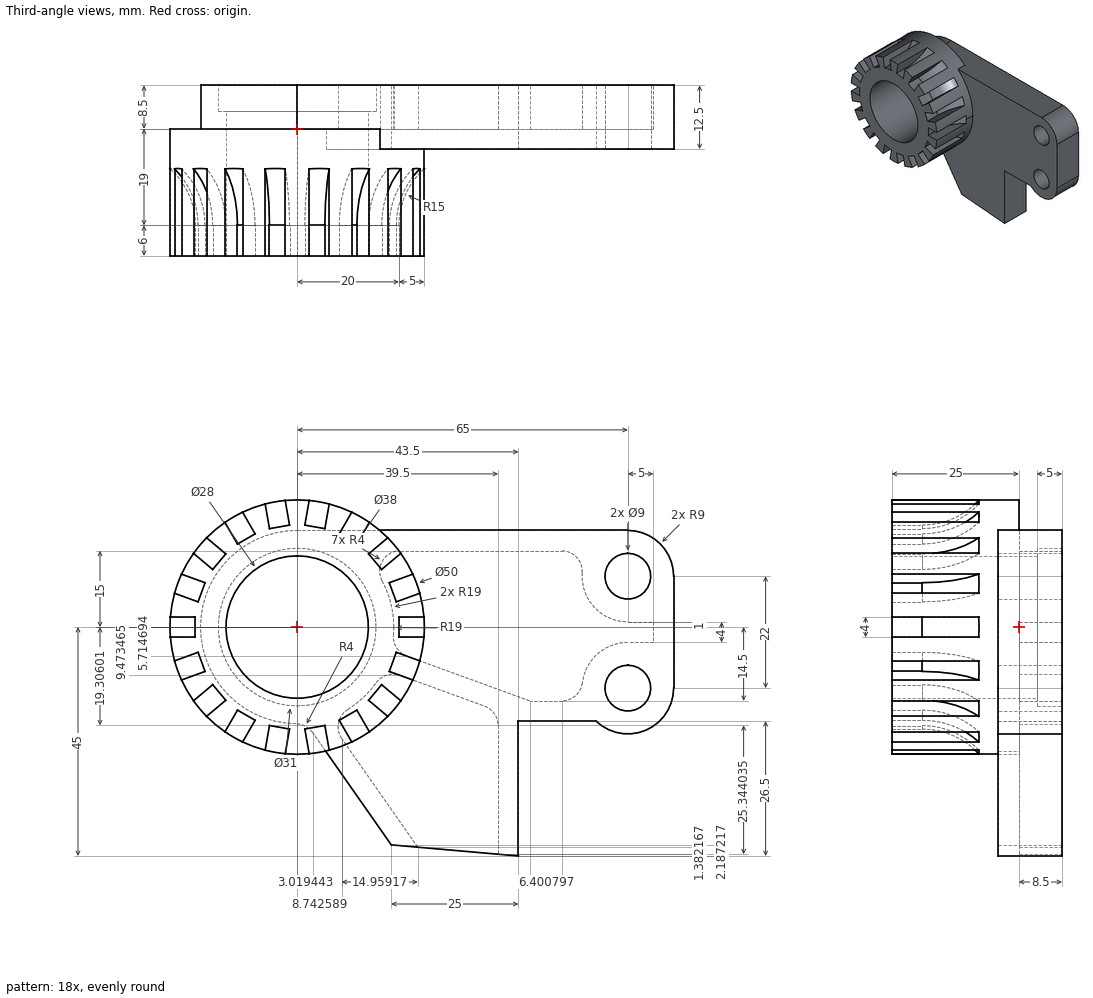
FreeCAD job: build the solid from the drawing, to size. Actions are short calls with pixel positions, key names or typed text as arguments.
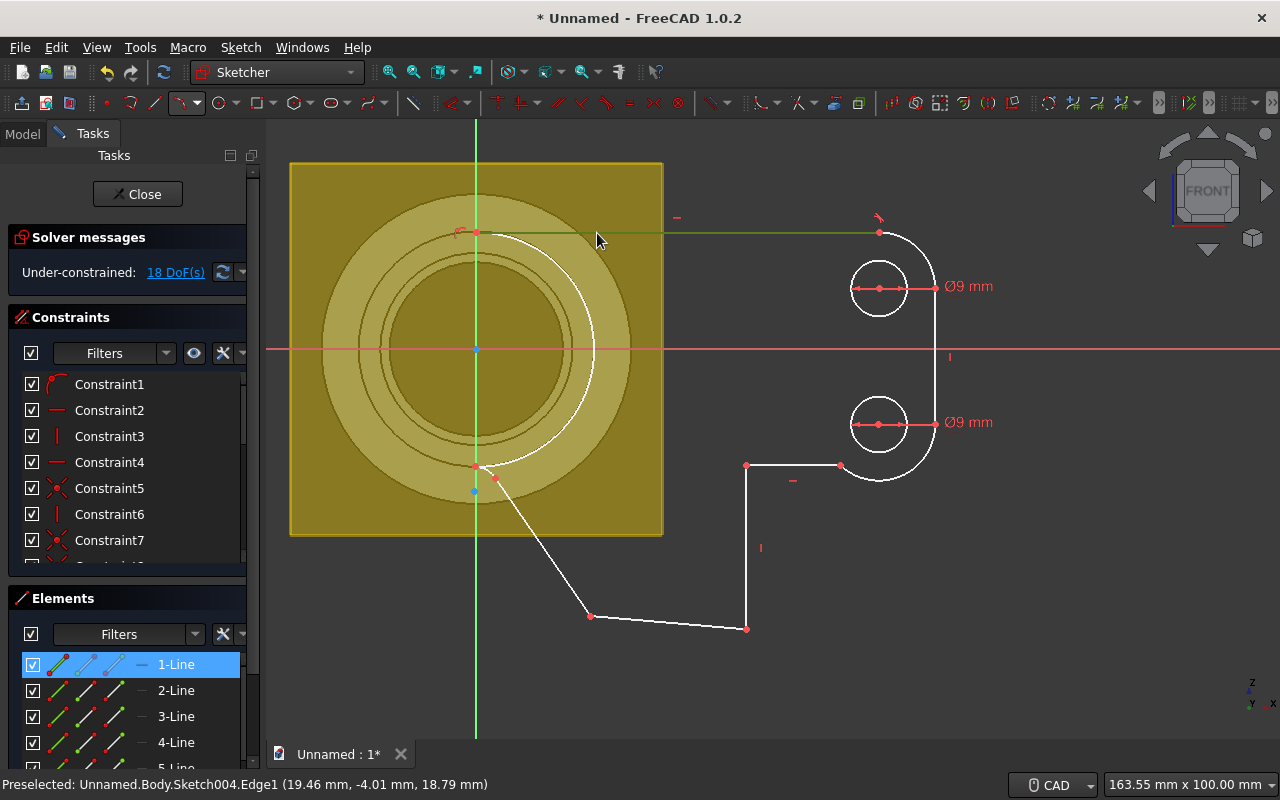
click(571, 420)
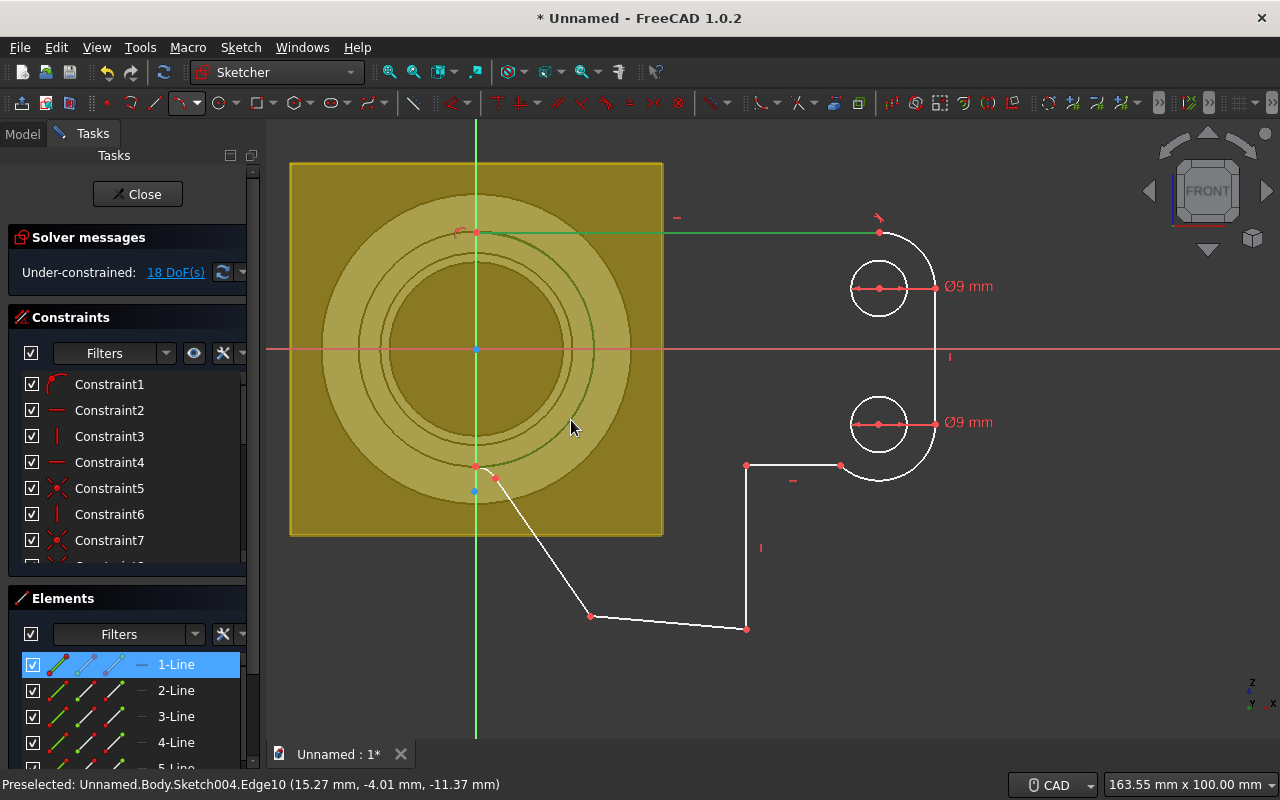
click(606, 104)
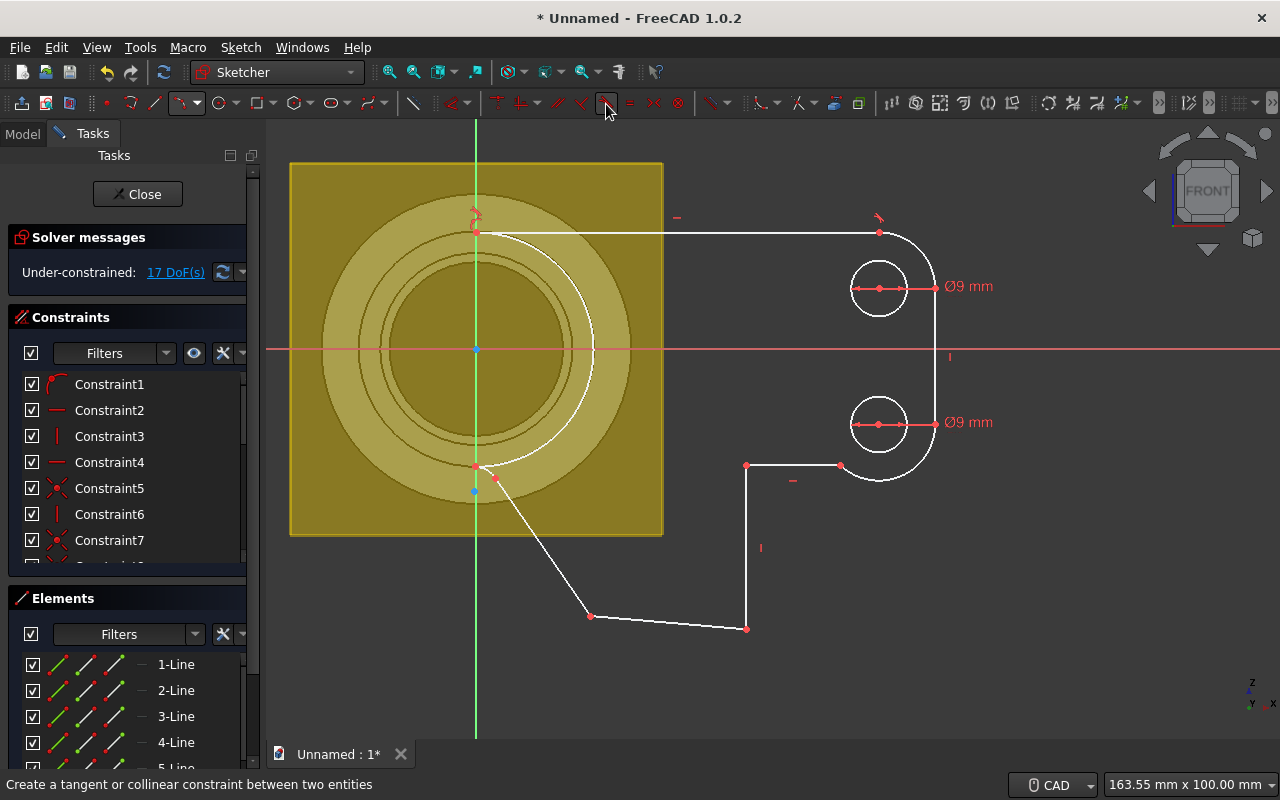
click(935, 329)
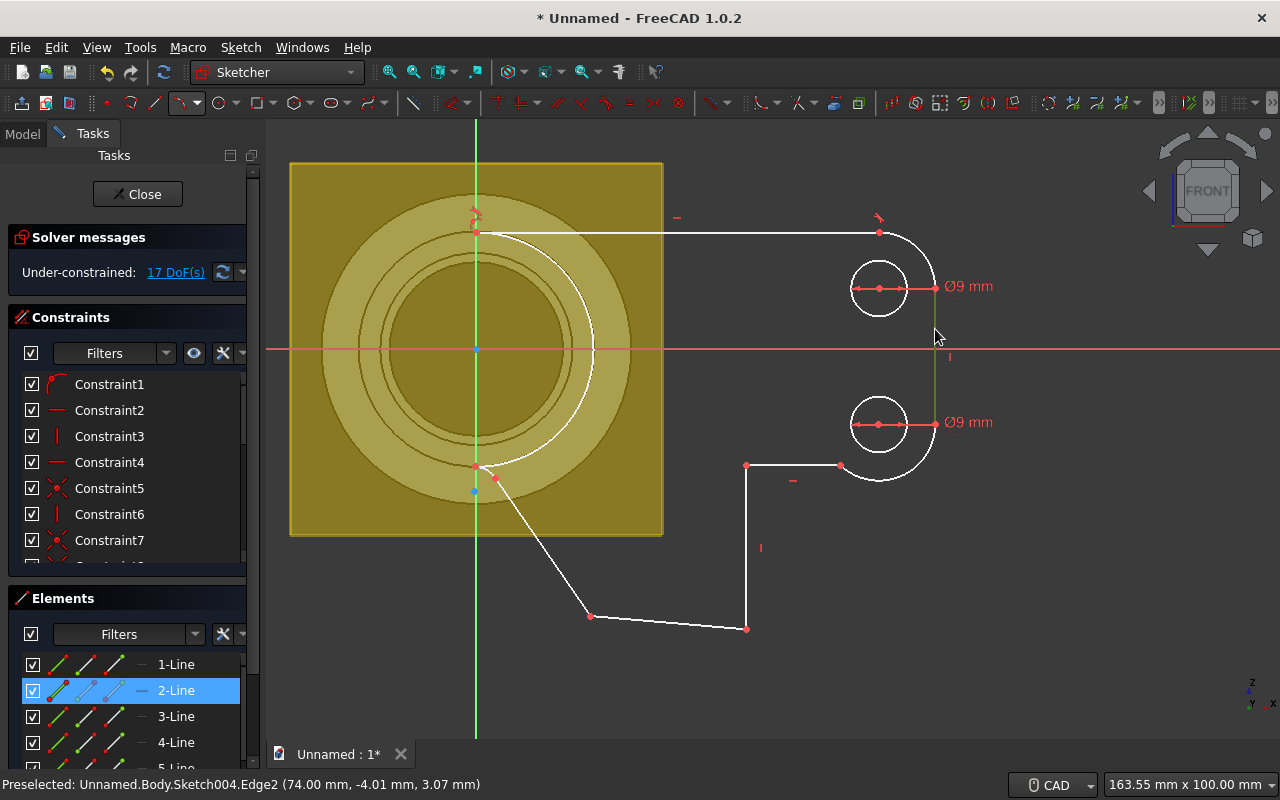
click(929, 263)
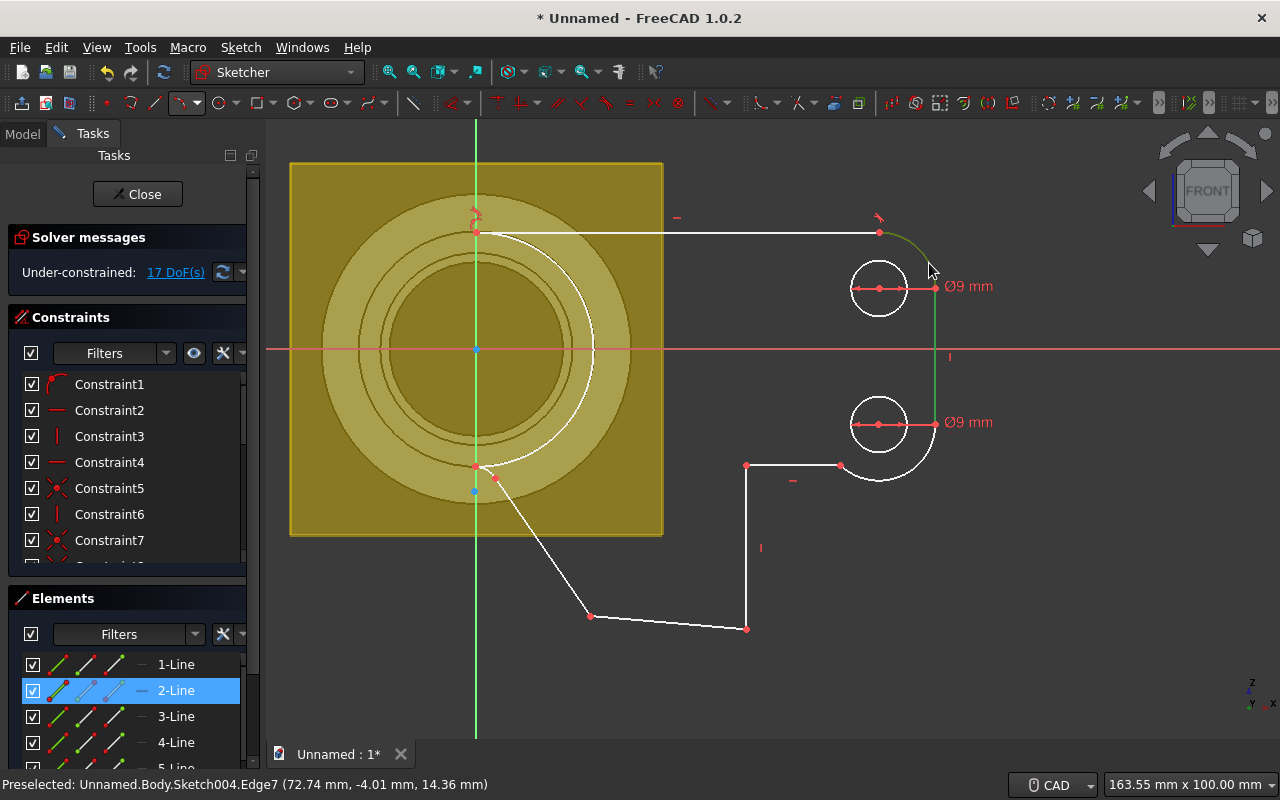
click(606, 104)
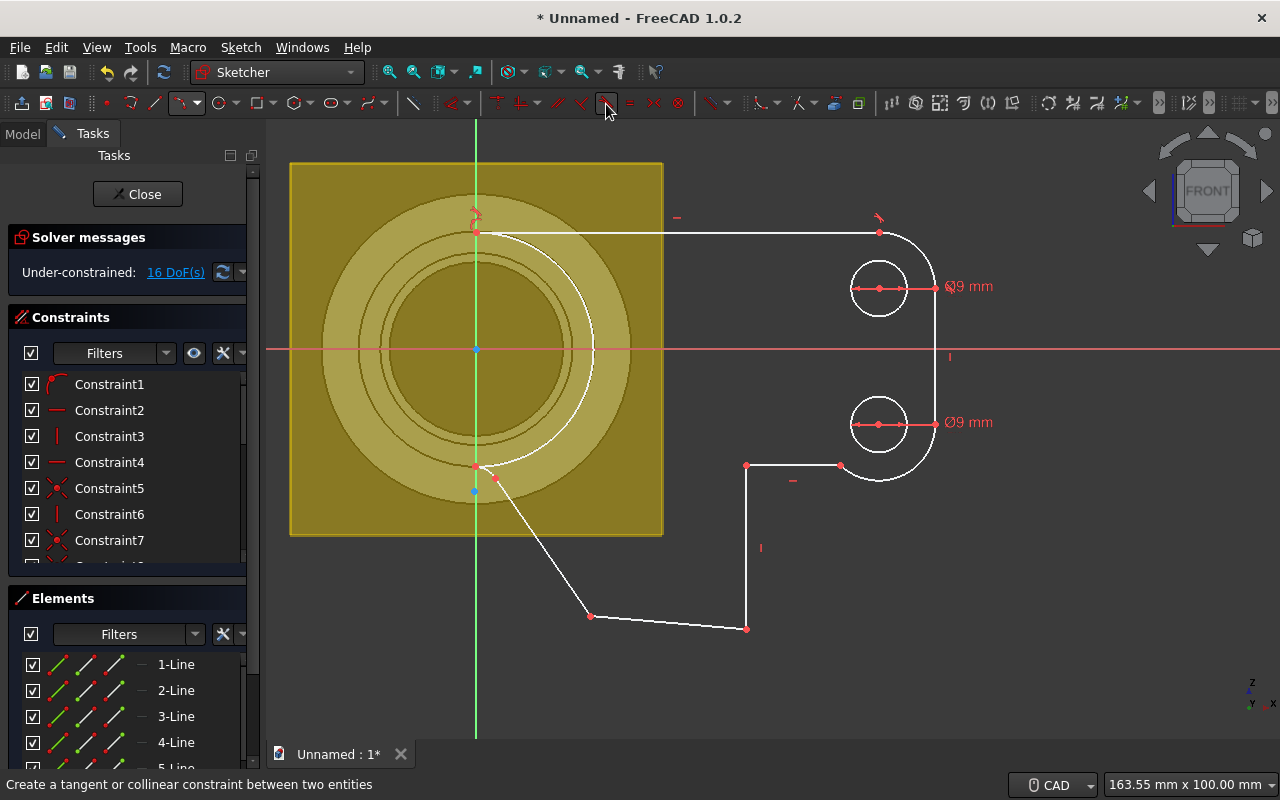
click(935, 329)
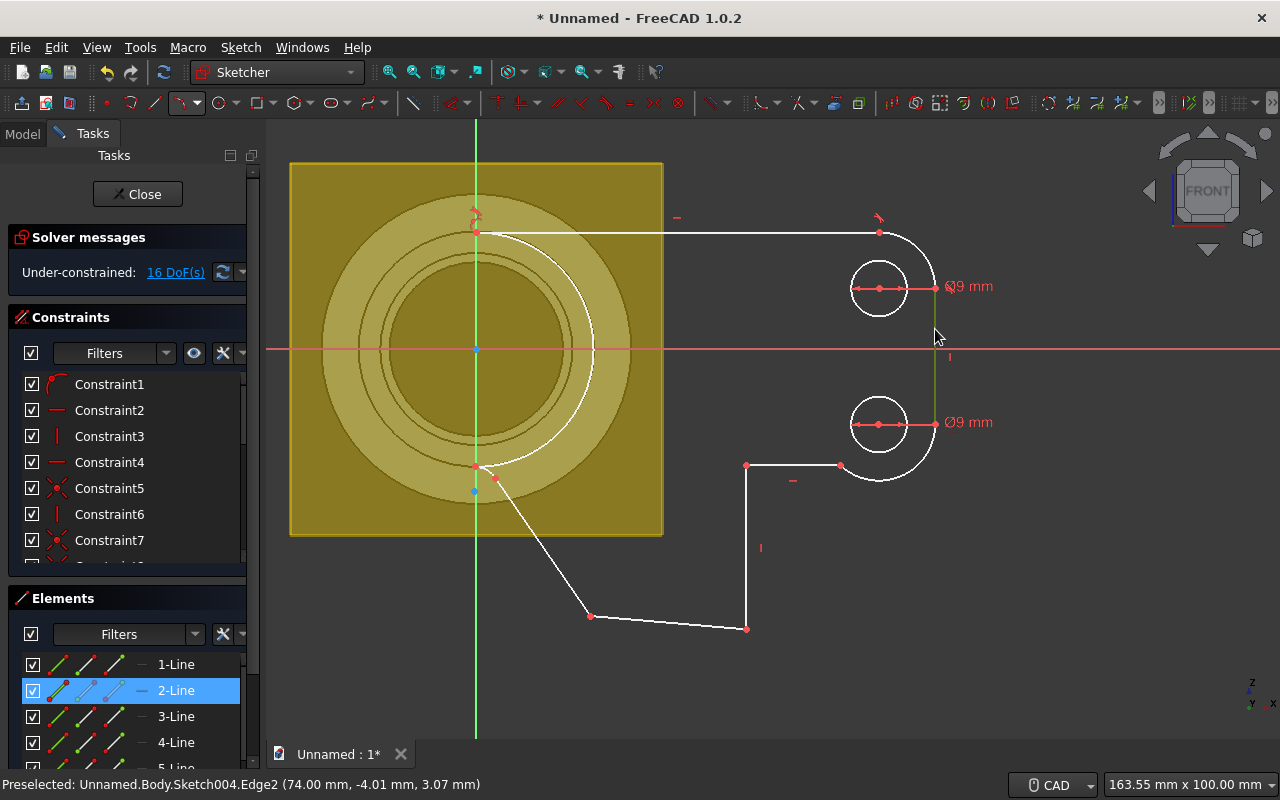
click(875, 481)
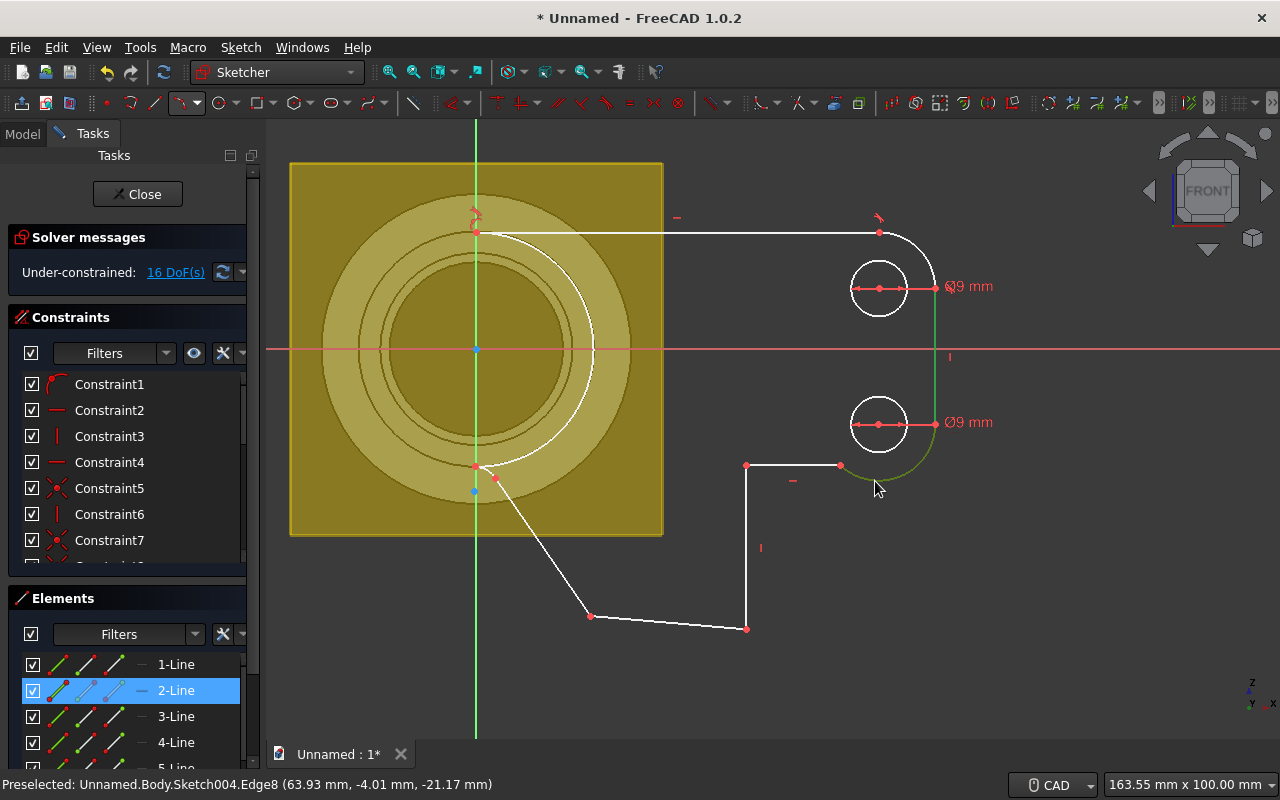
click(606, 104)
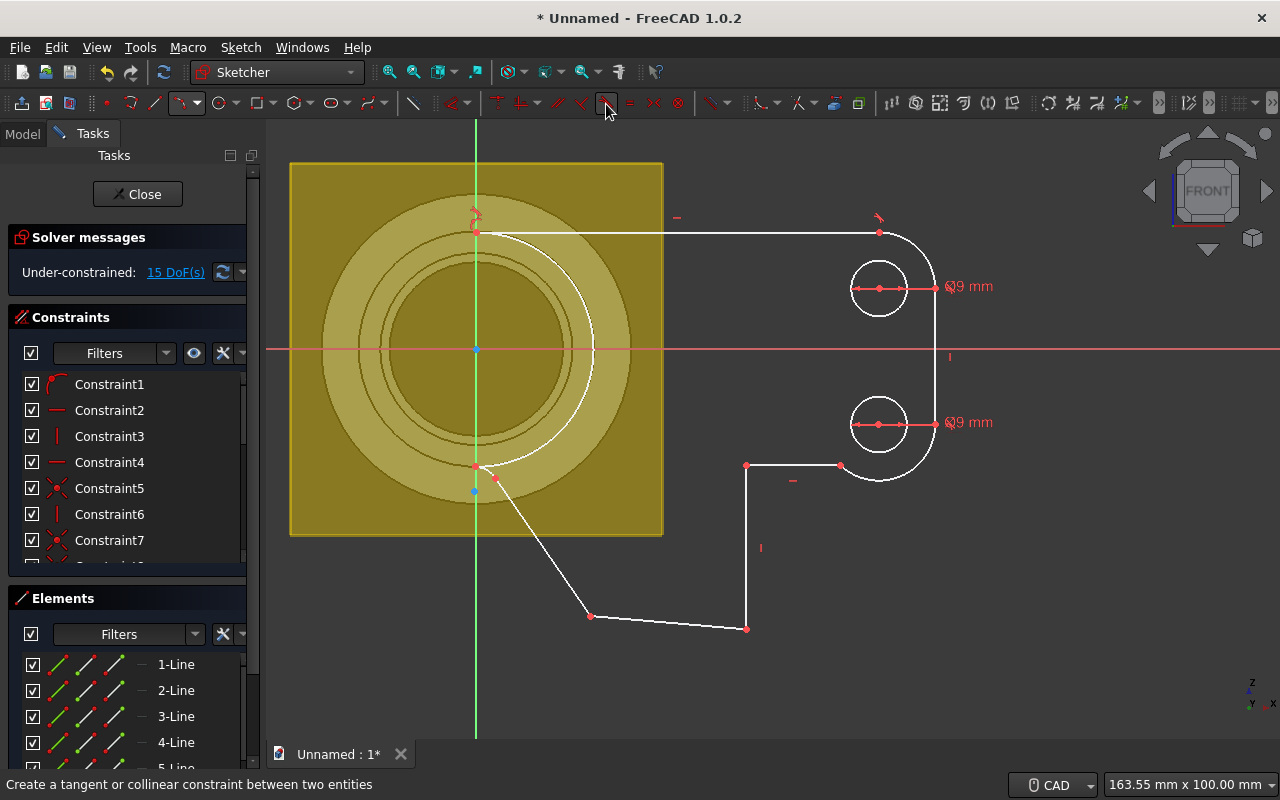
click(562, 575)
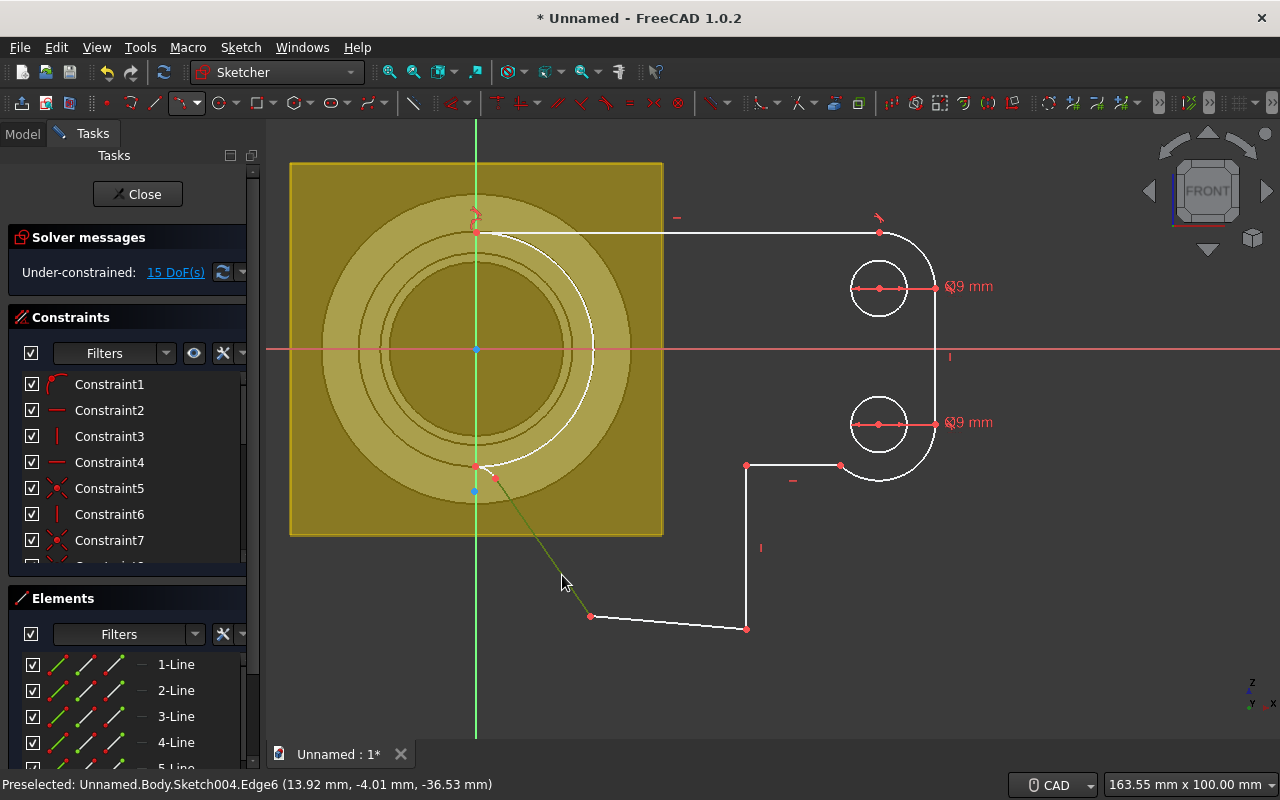
scroll(491, 473, up, 4)